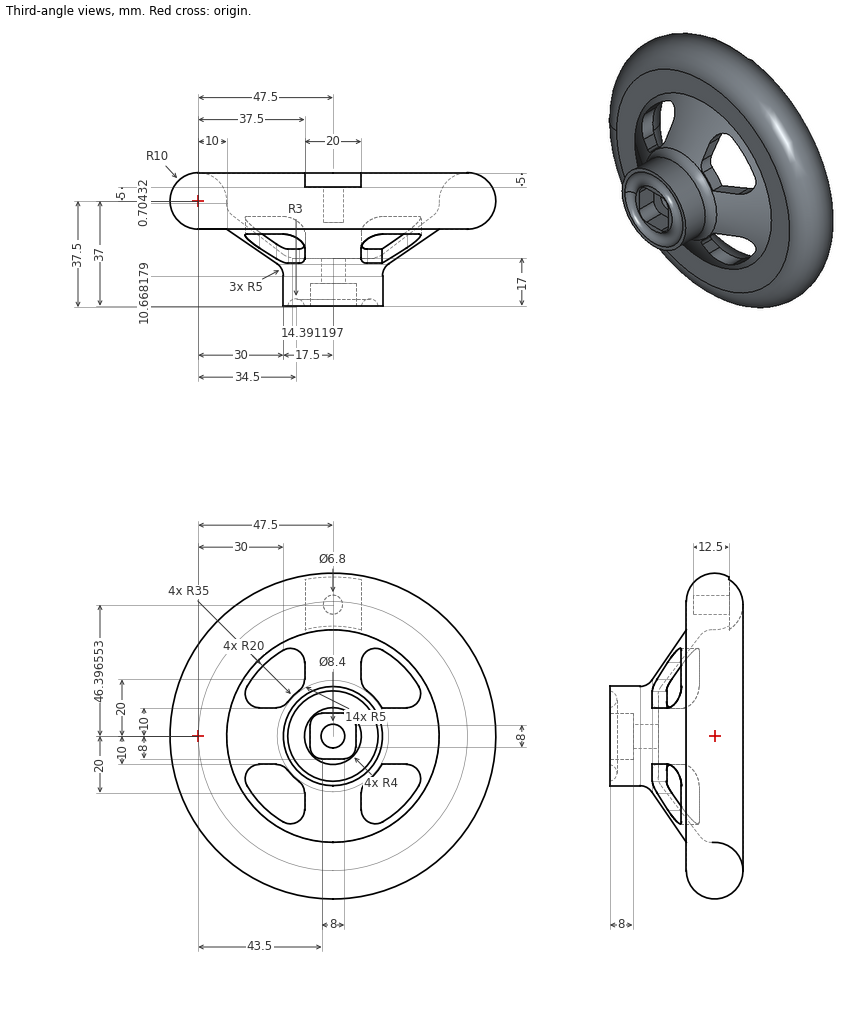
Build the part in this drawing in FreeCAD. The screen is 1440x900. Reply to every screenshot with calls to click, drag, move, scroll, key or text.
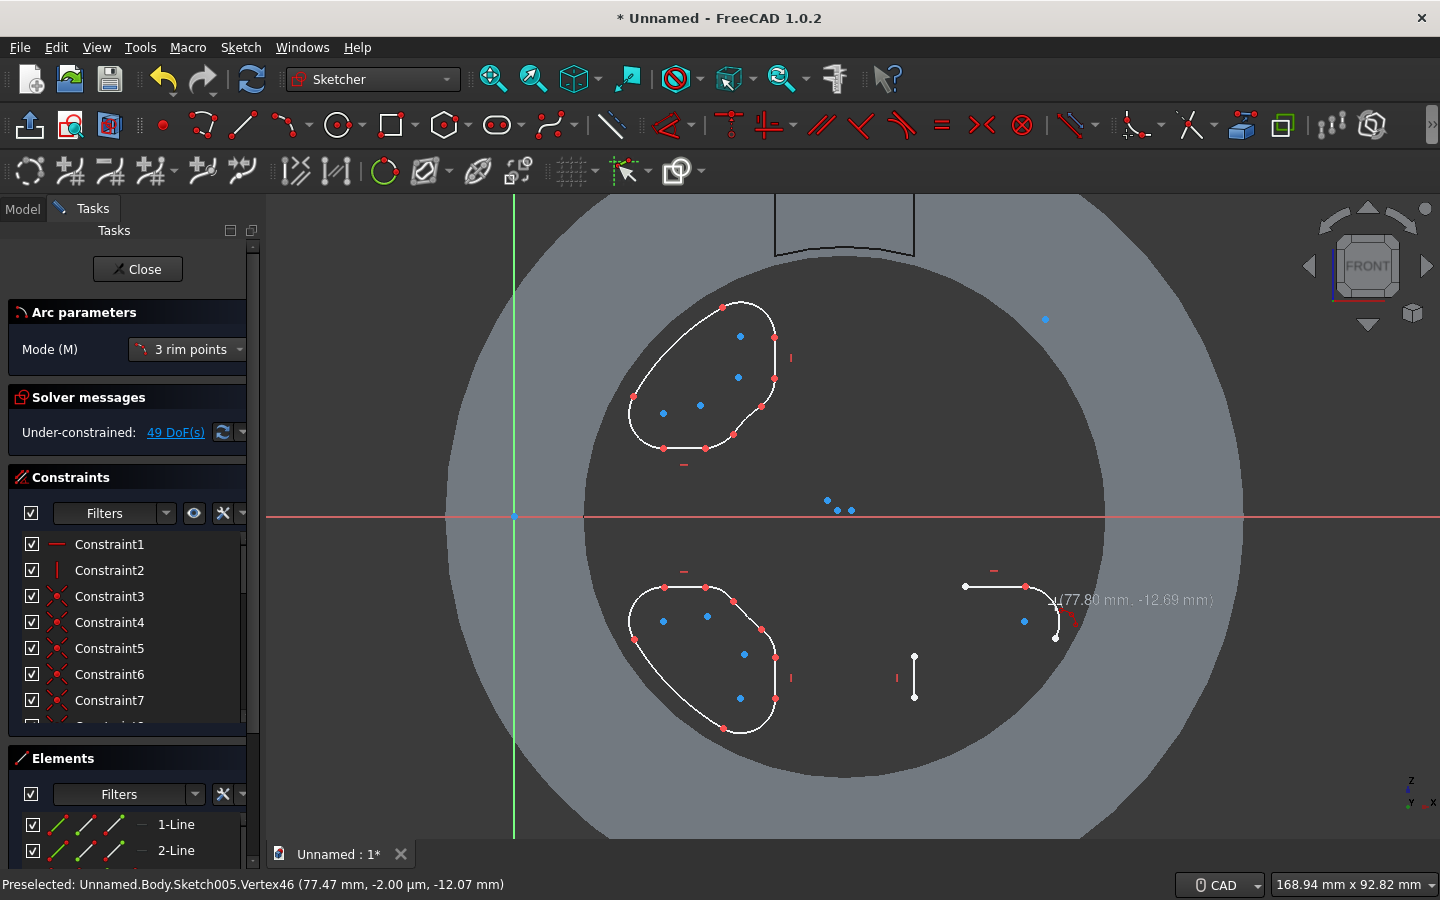
click(1055, 639)
click(966, 727)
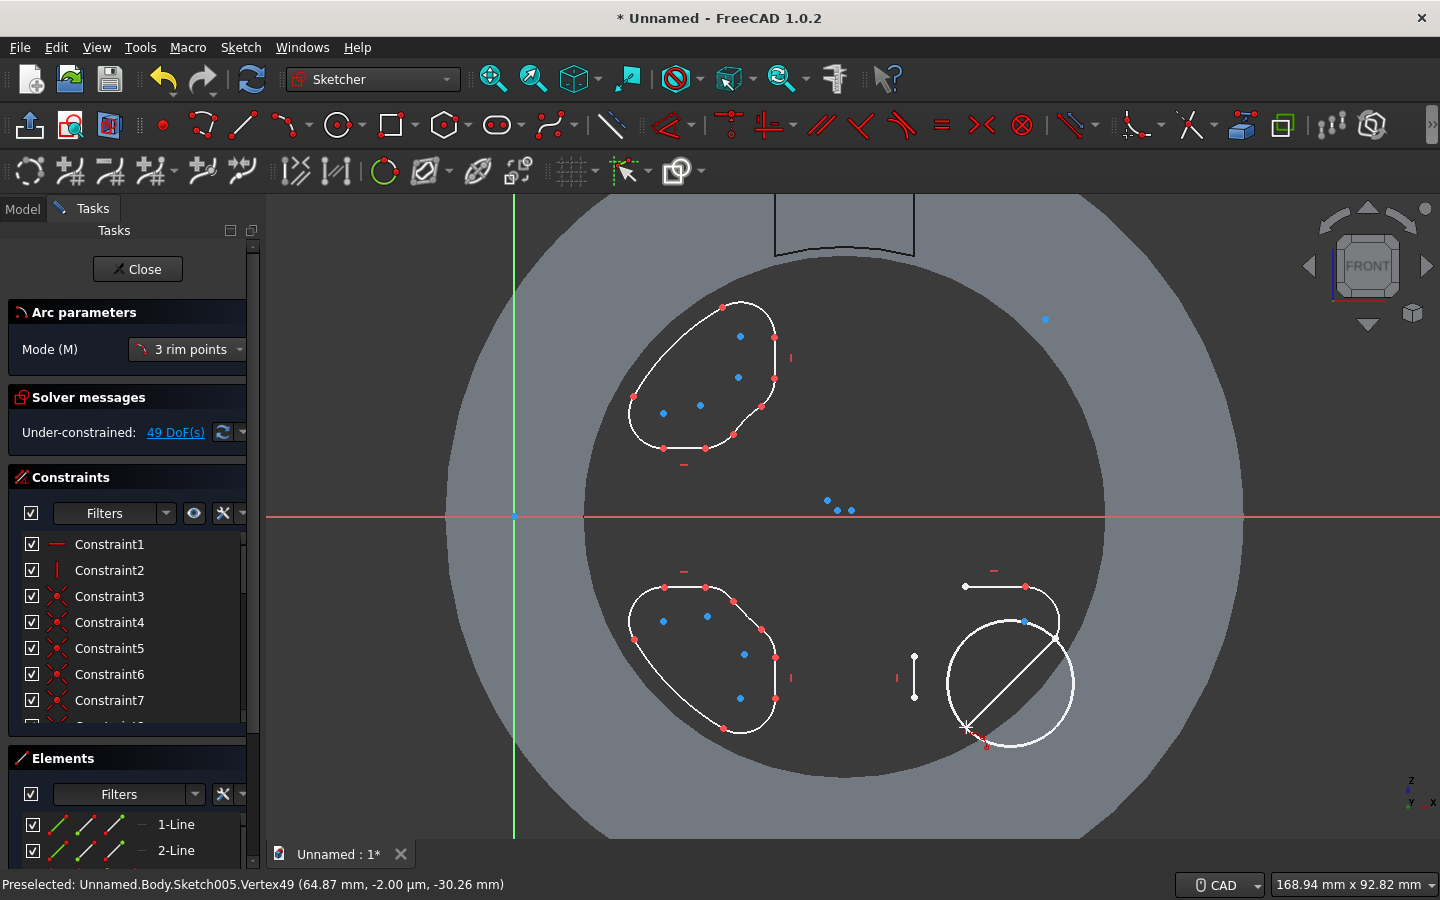
scroll(1016, 689, up, 4)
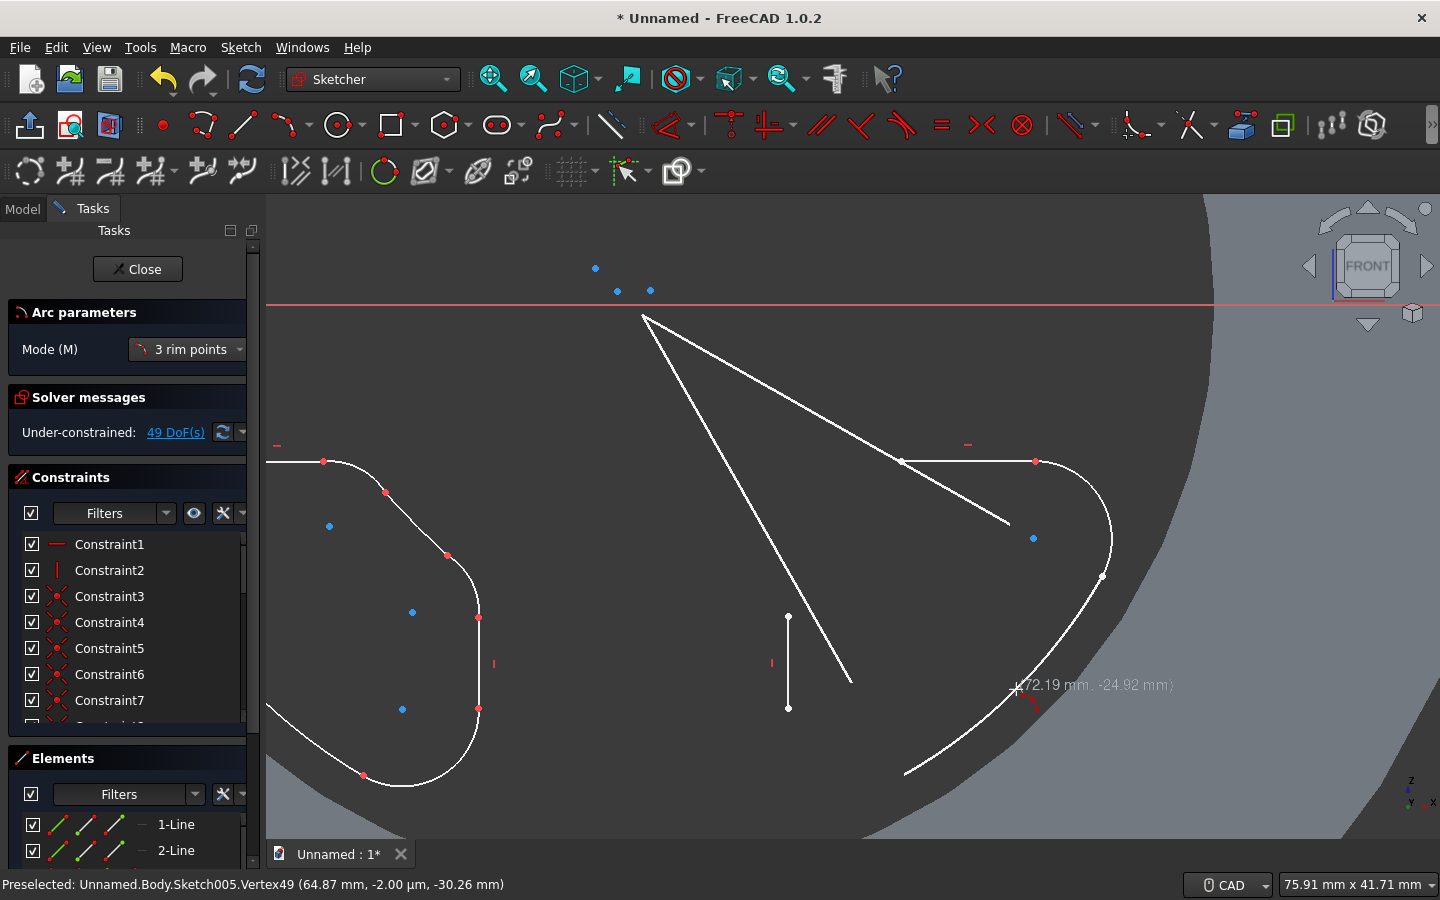
click(1016, 688)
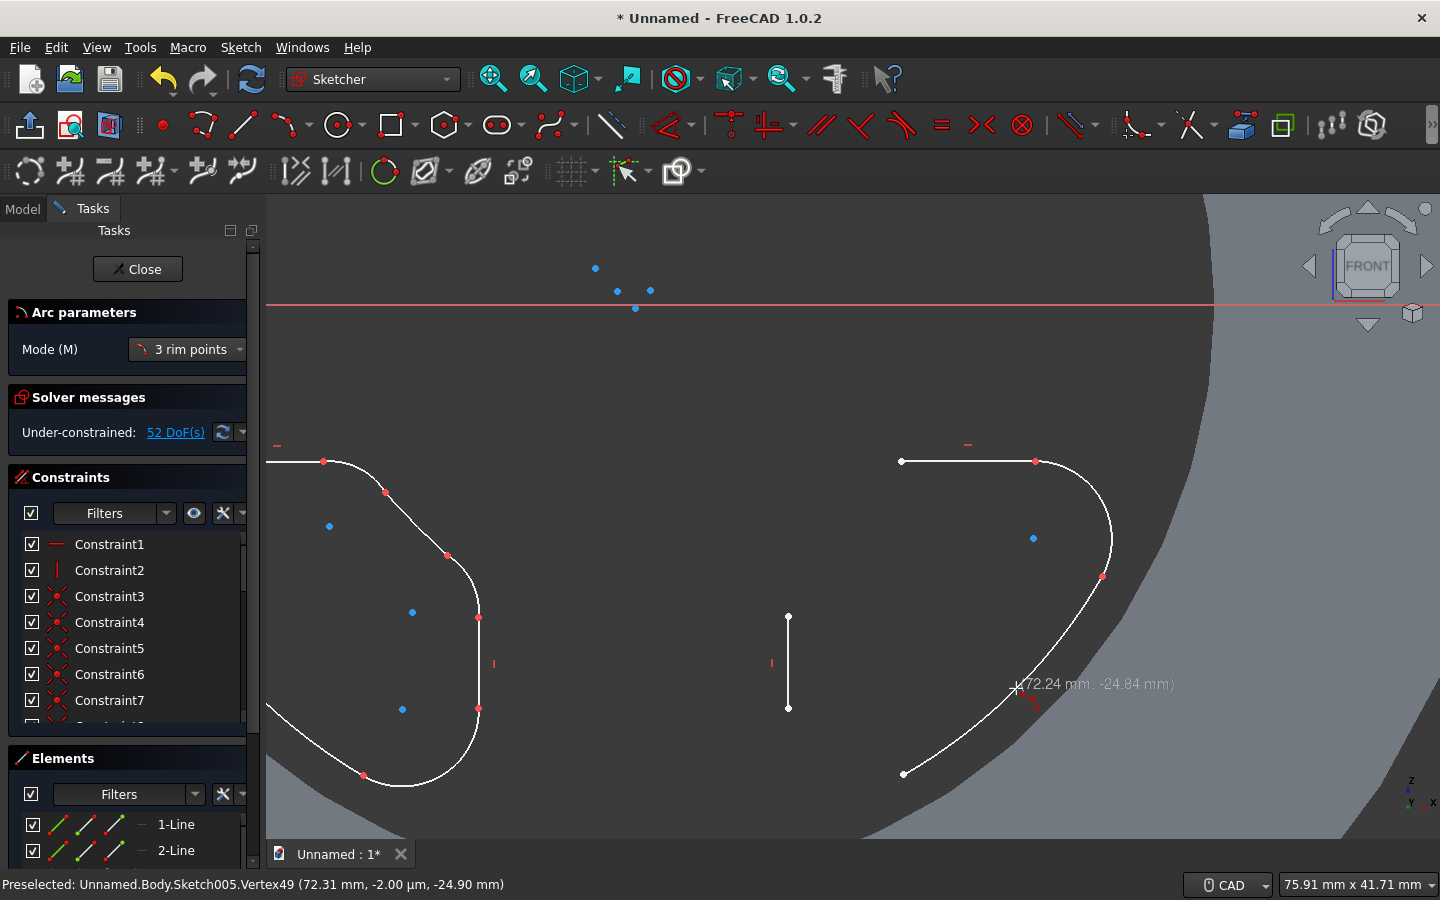
click(904, 775)
click(788, 708)
click(827, 774)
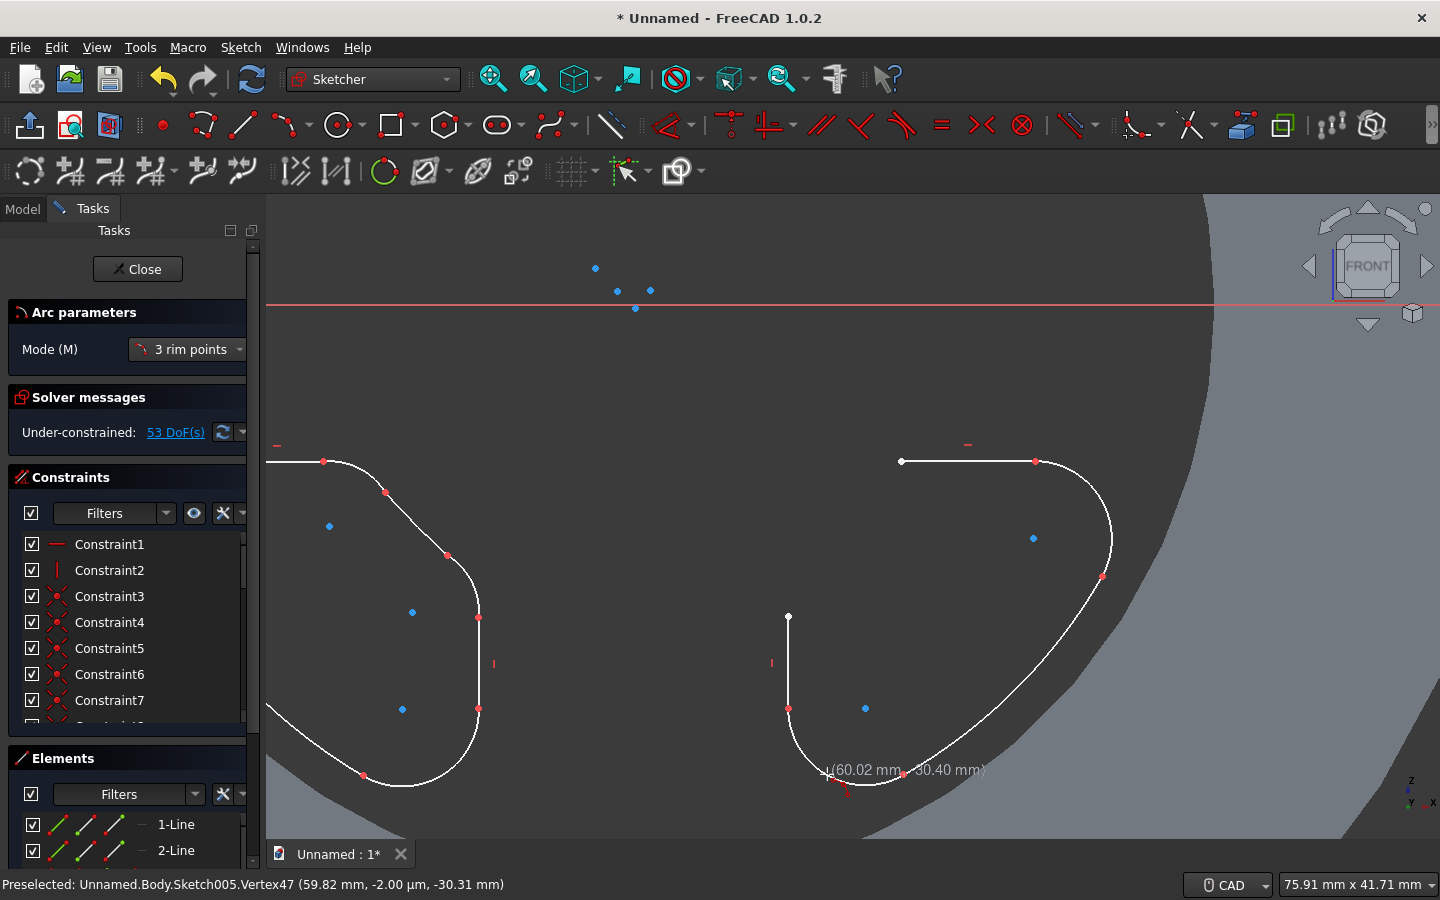
click(788, 617)
click(819, 552)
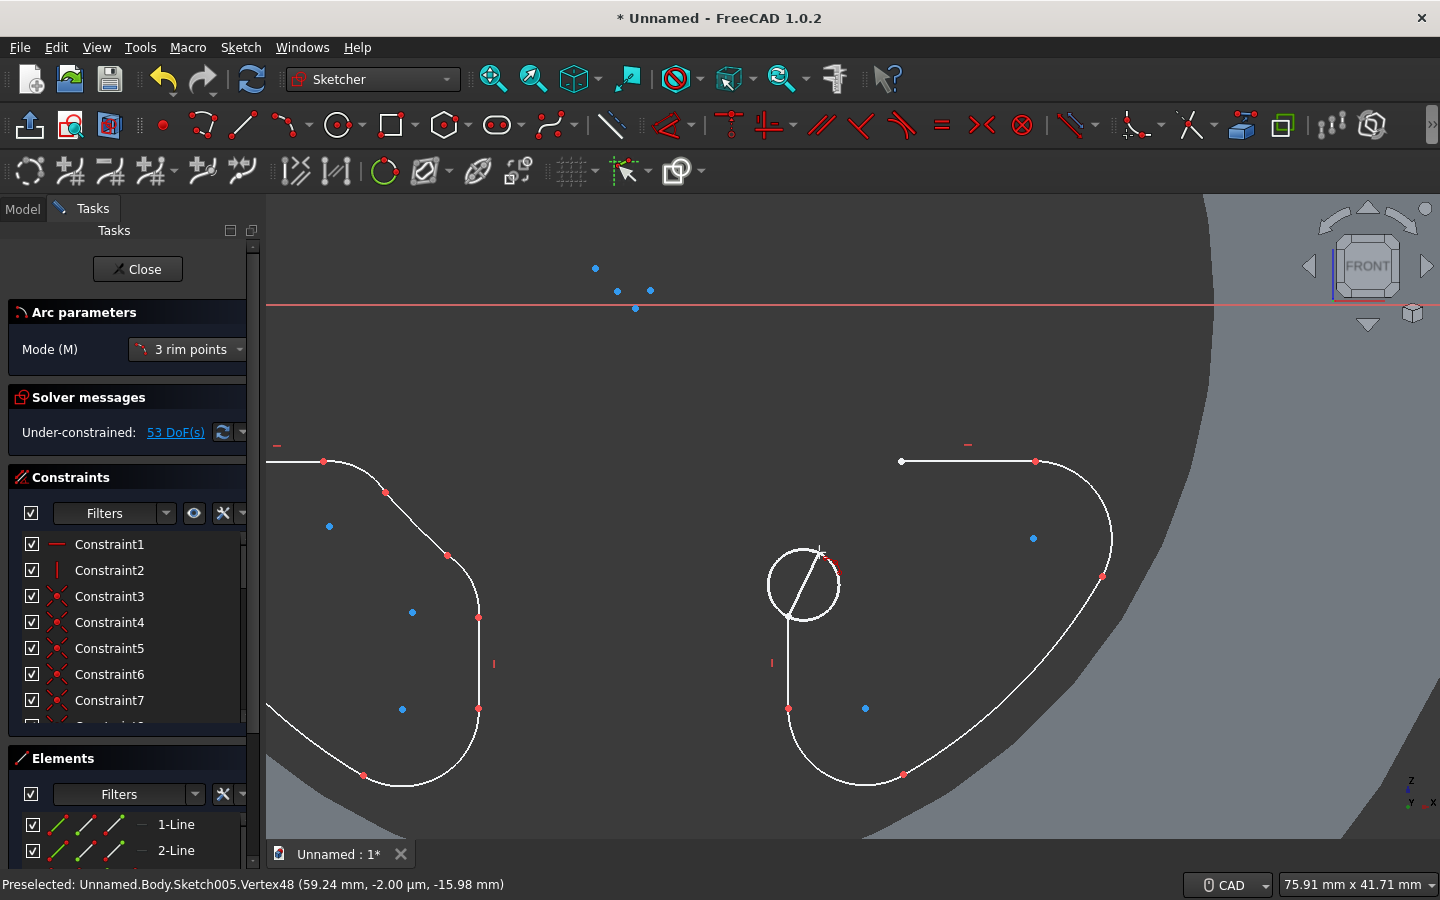
scroll(796, 580, up, 4)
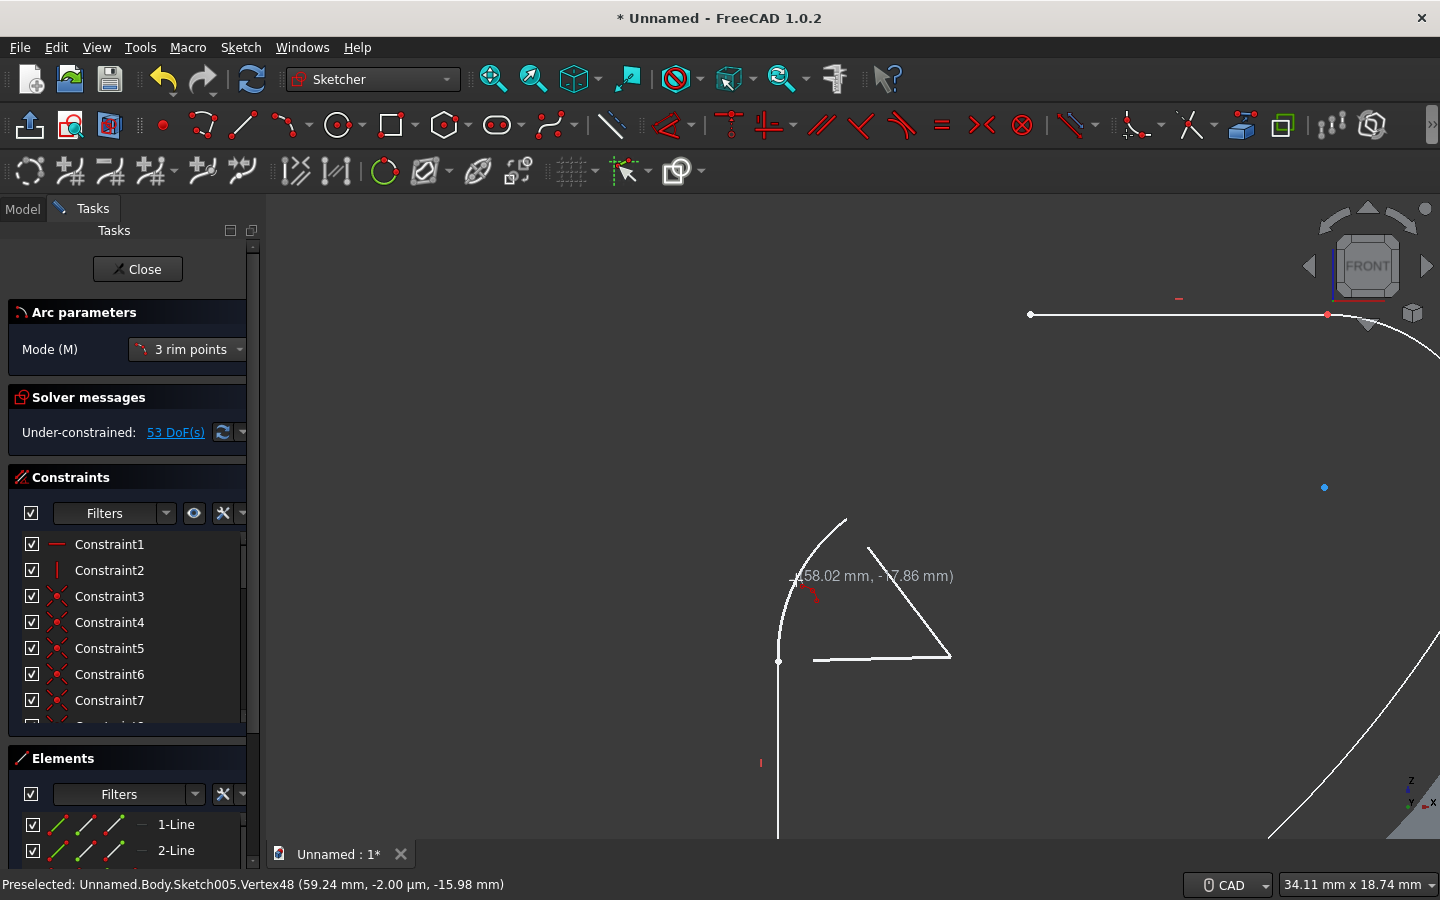
click(796, 578)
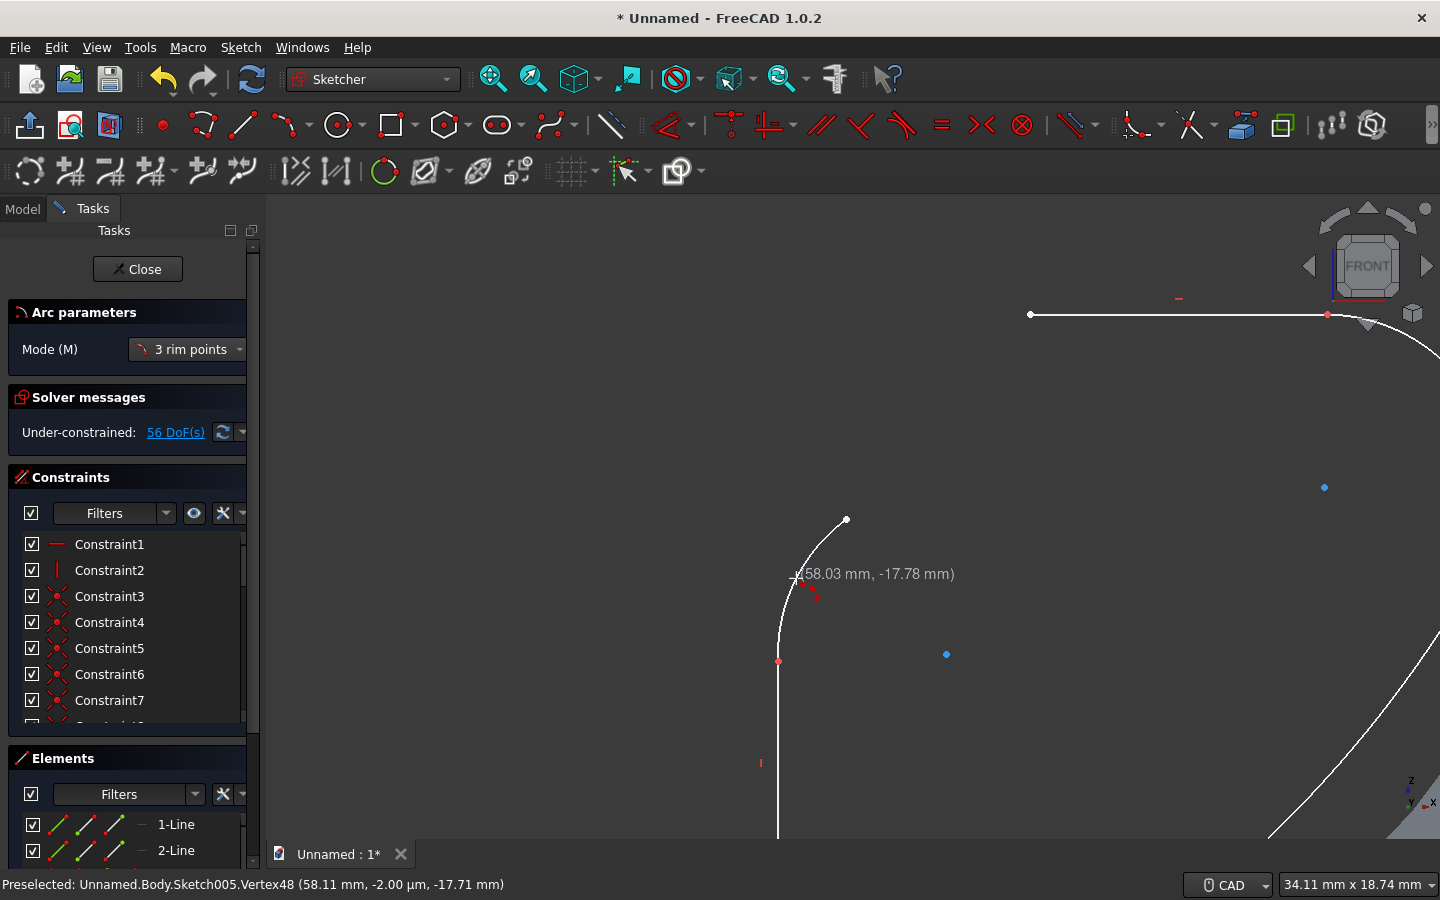
scroll(948, 656, down, 8)